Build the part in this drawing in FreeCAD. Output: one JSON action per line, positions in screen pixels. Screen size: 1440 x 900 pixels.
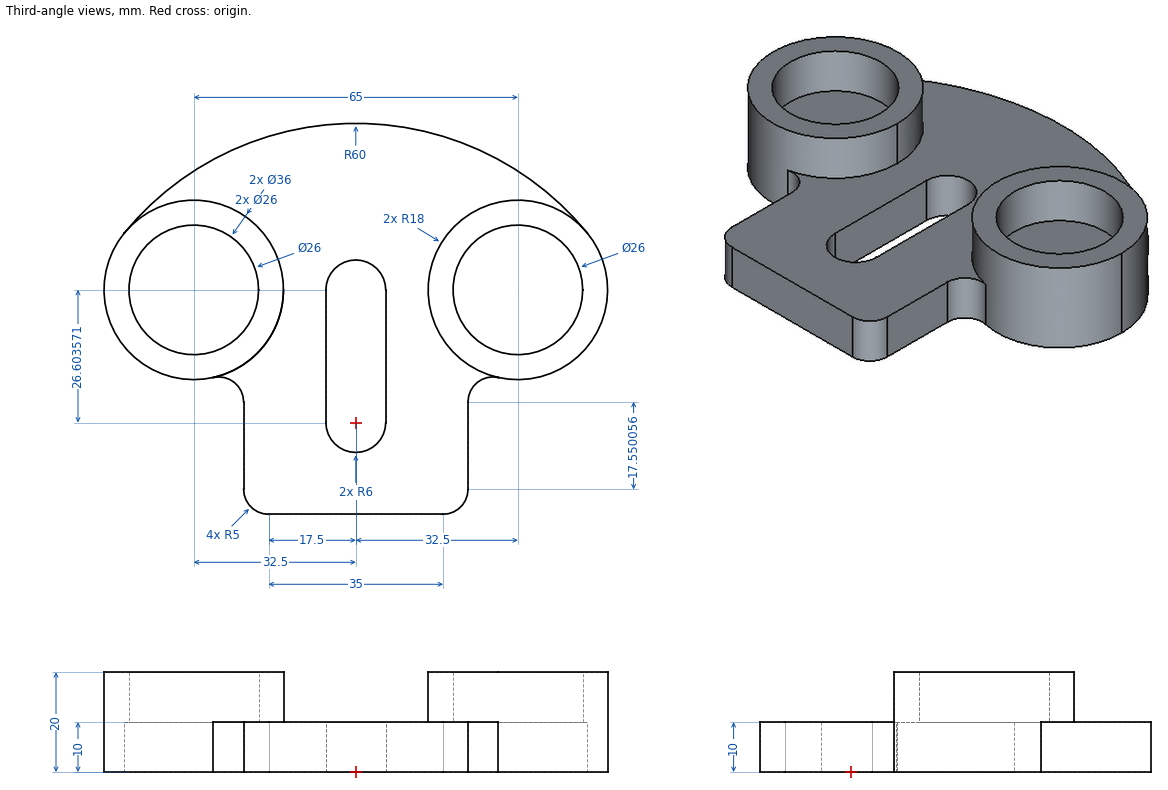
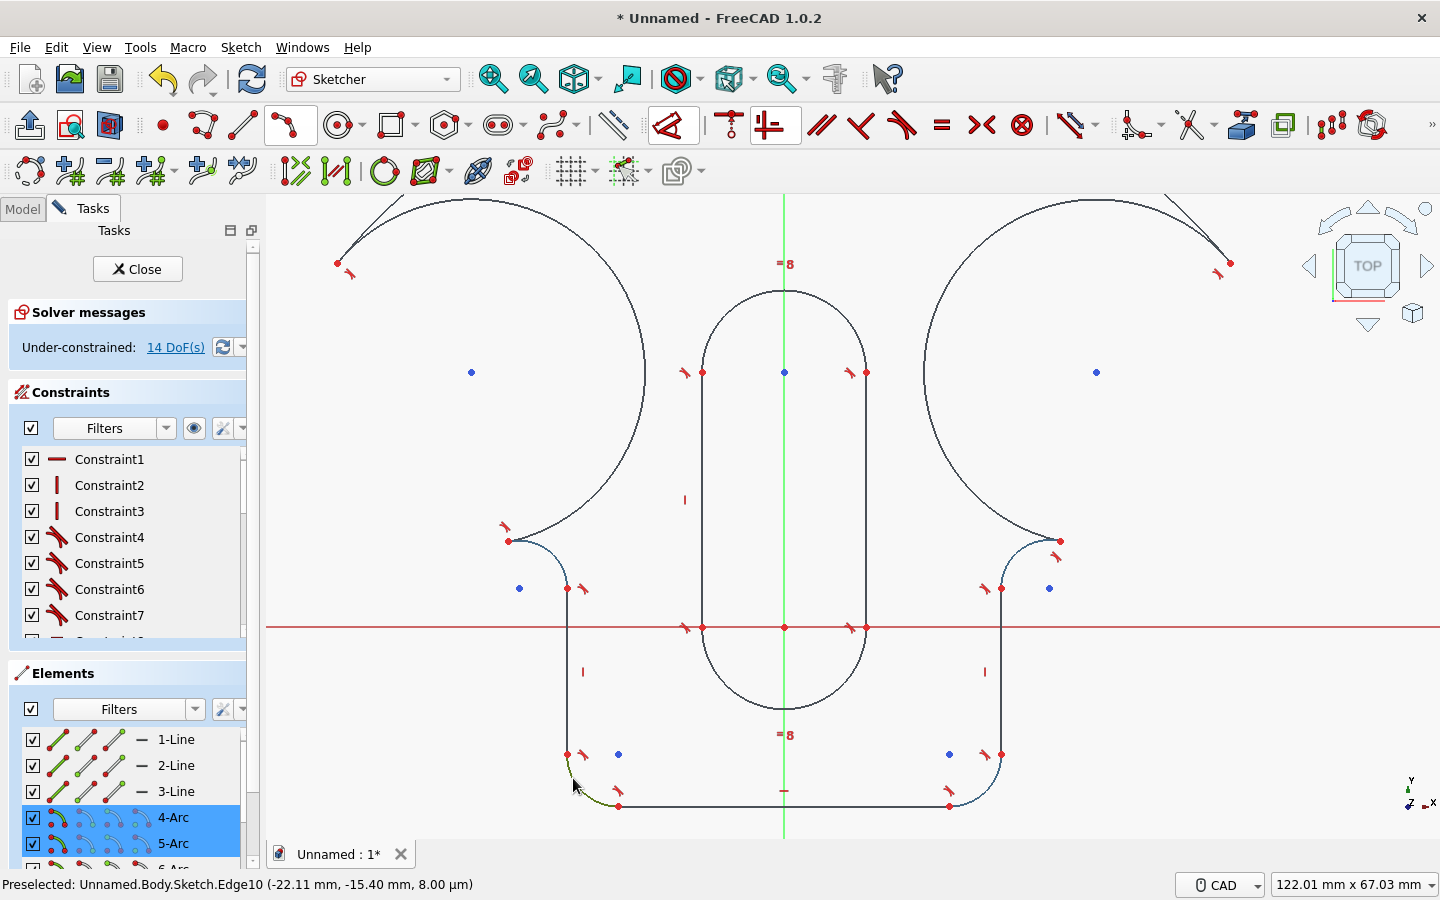
{"action": "left_click", "coordinate": [942, 126]}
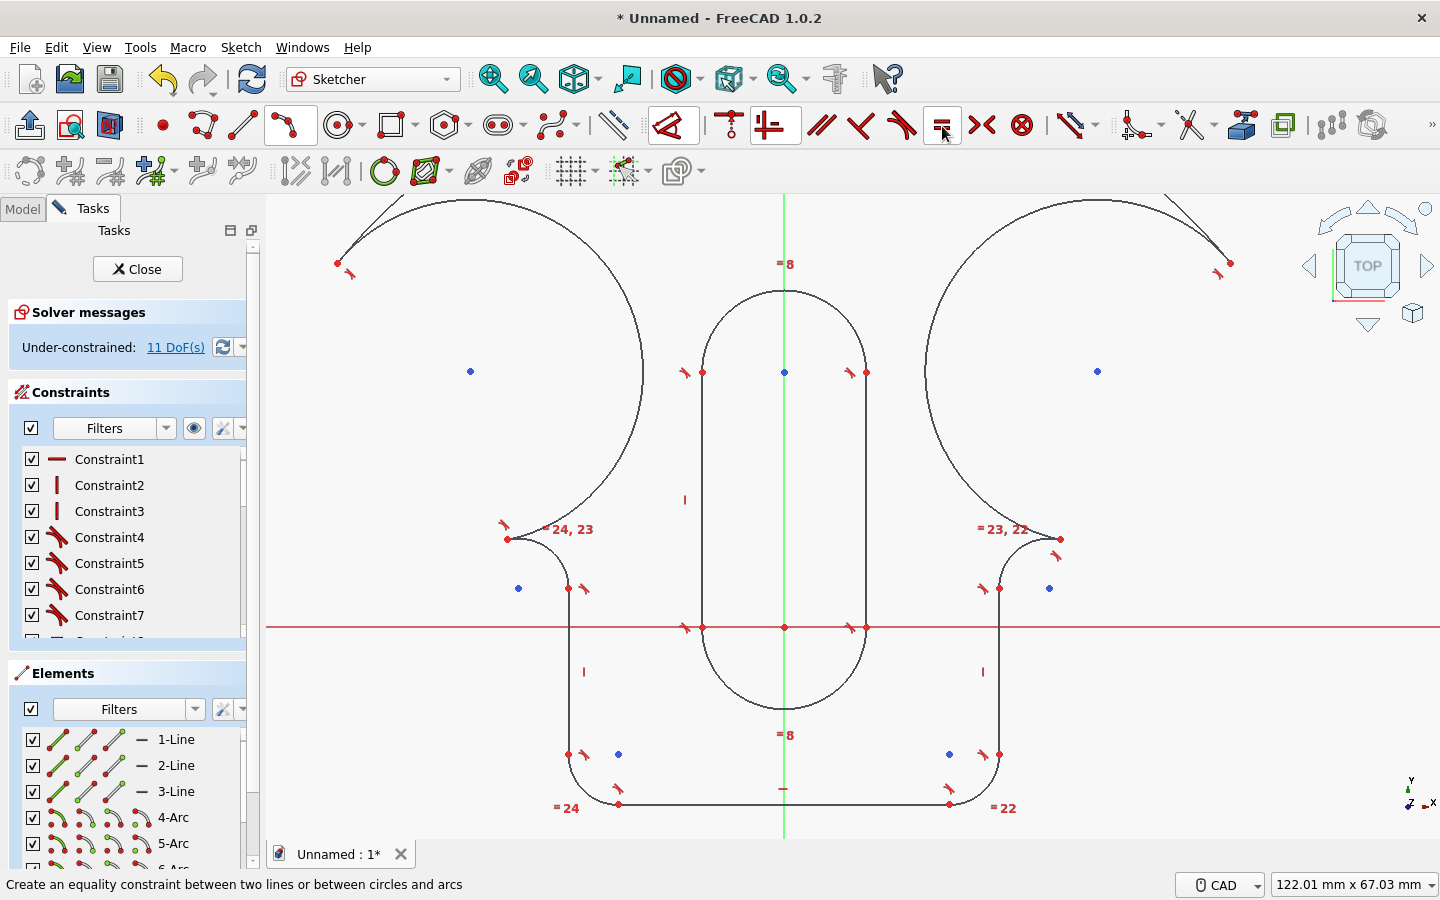
{"action": "left_click", "coordinate": [929, 408]}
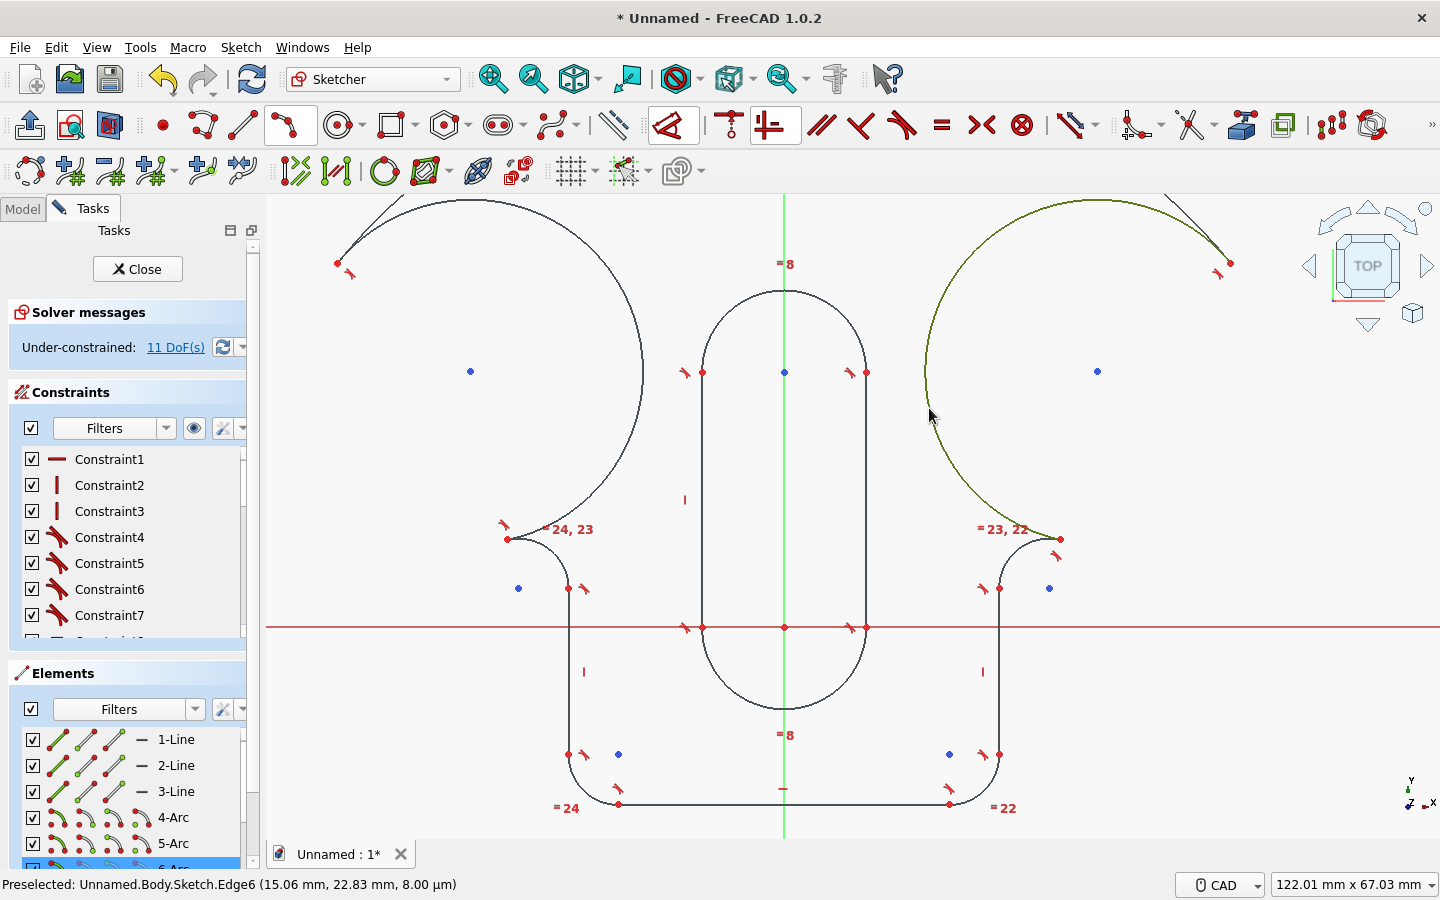
{"action": "left_click", "coordinate": [639, 408]}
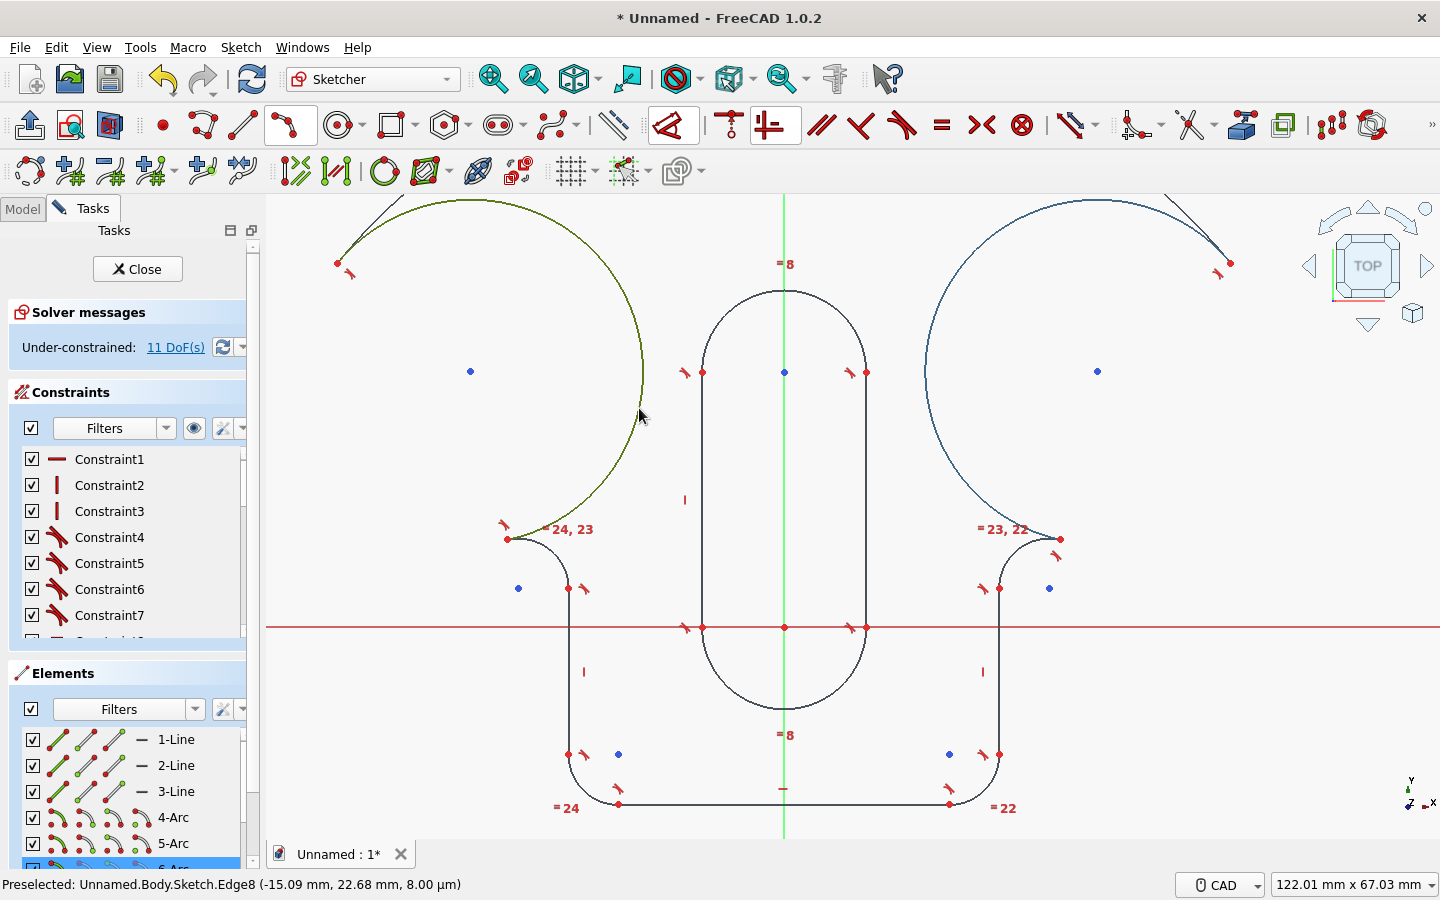
{"action": "left_click", "coordinate": [942, 126]}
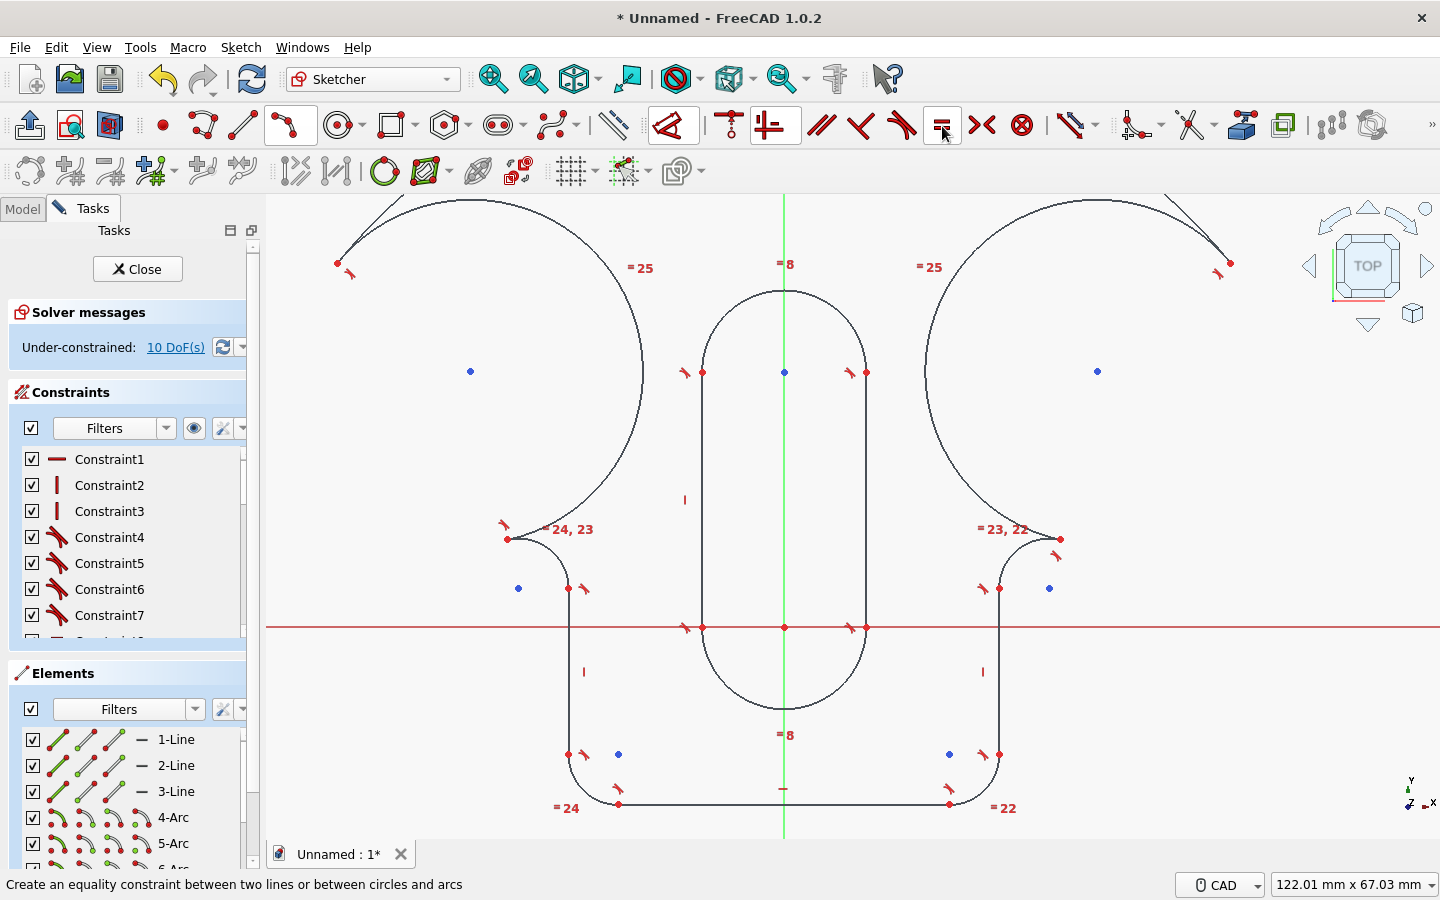
{"action": "left_click", "coordinate": [668, 126]}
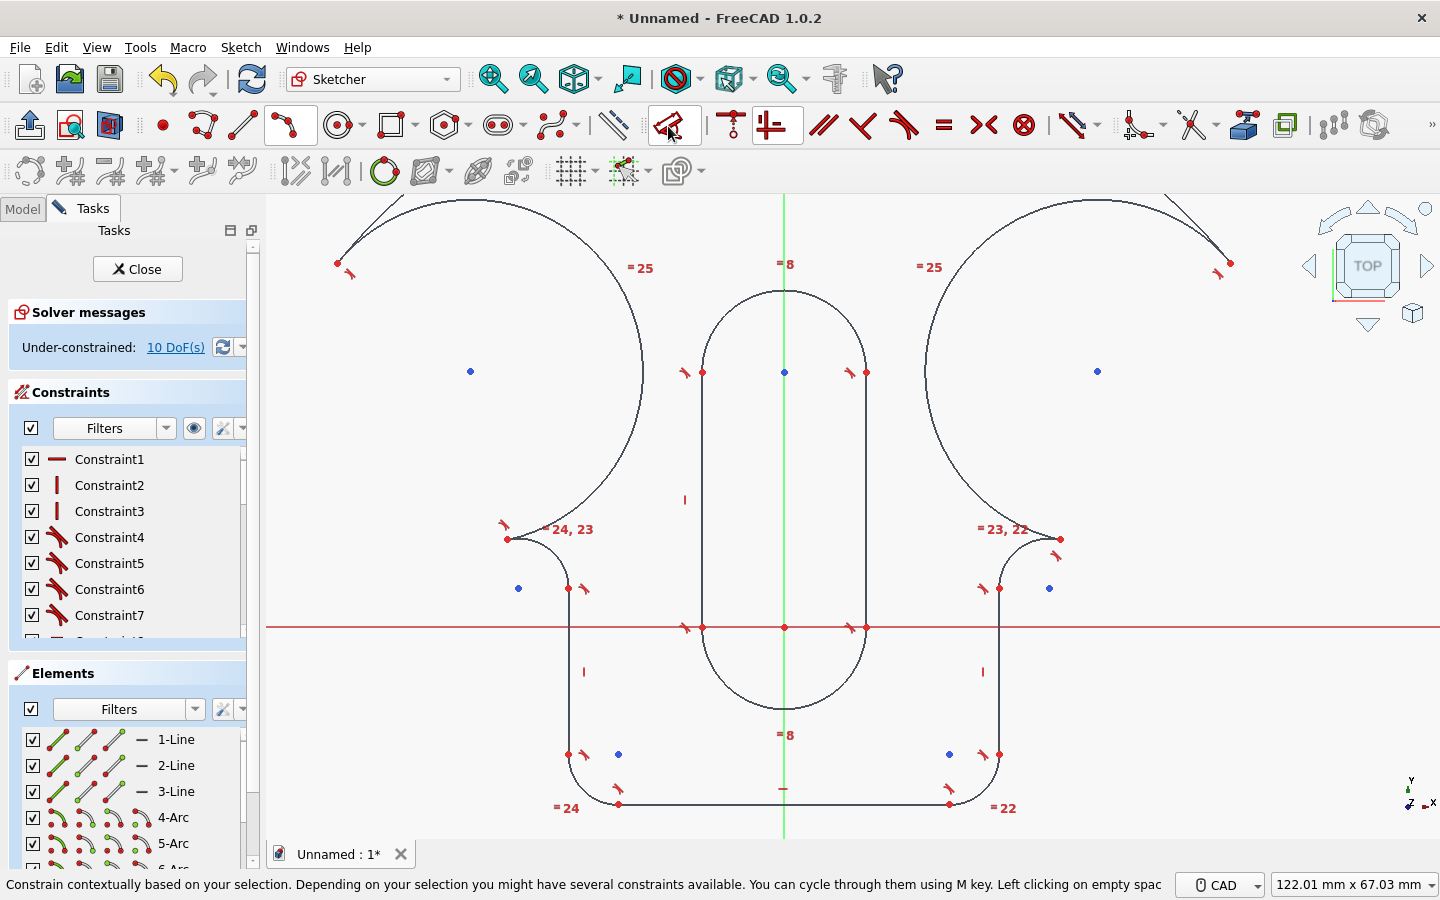
{"action": "left_click", "coordinate": [972, 799]}
{"action": "left_click", "coordinate": [1017, 800]}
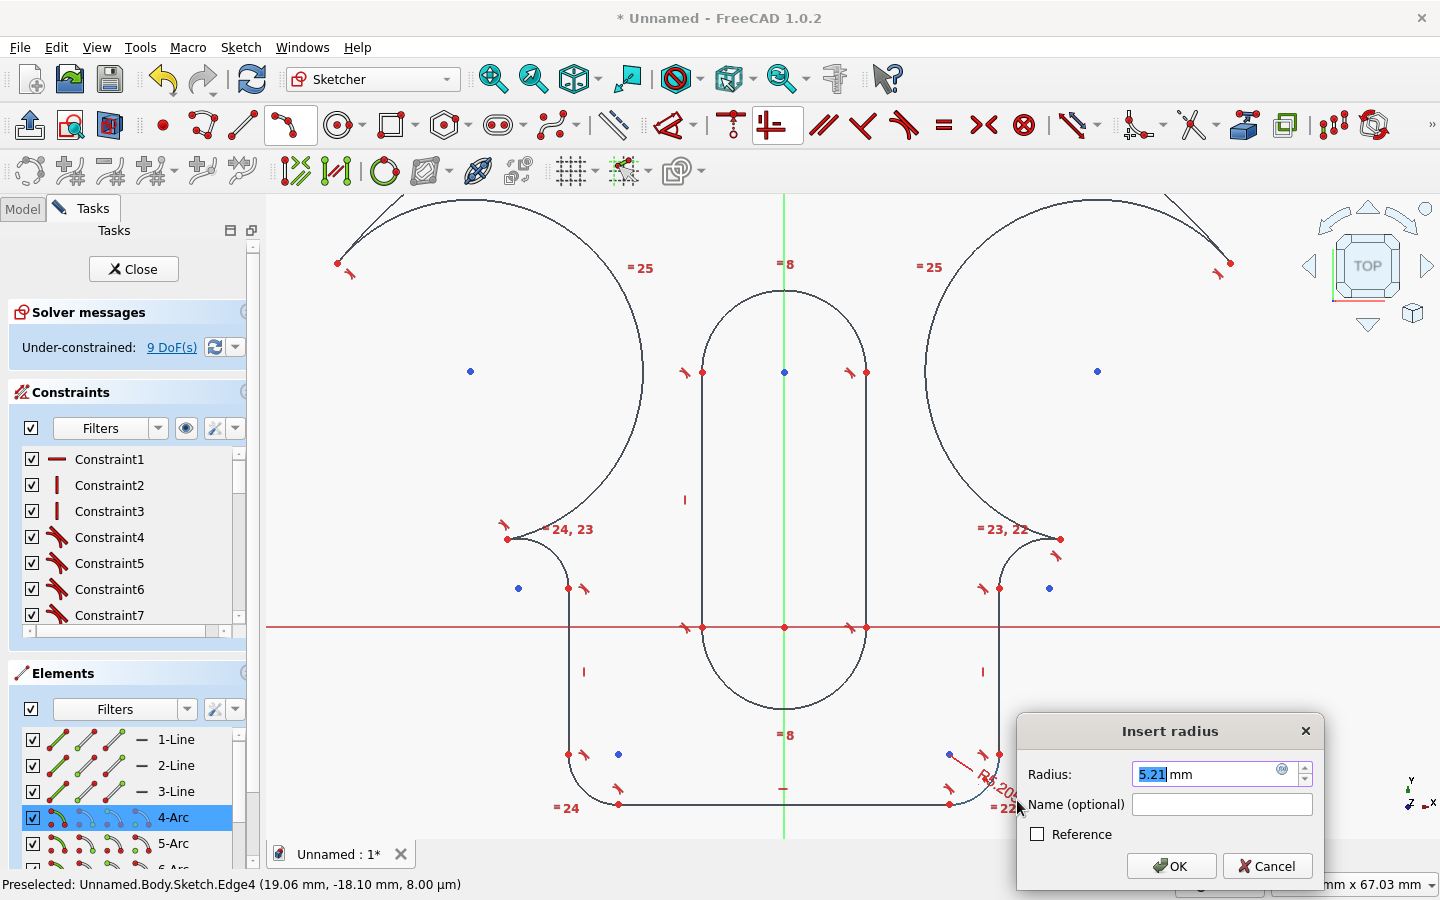
{"action": "type", "text": "5"}
{"action": "key", "text": "Return"}